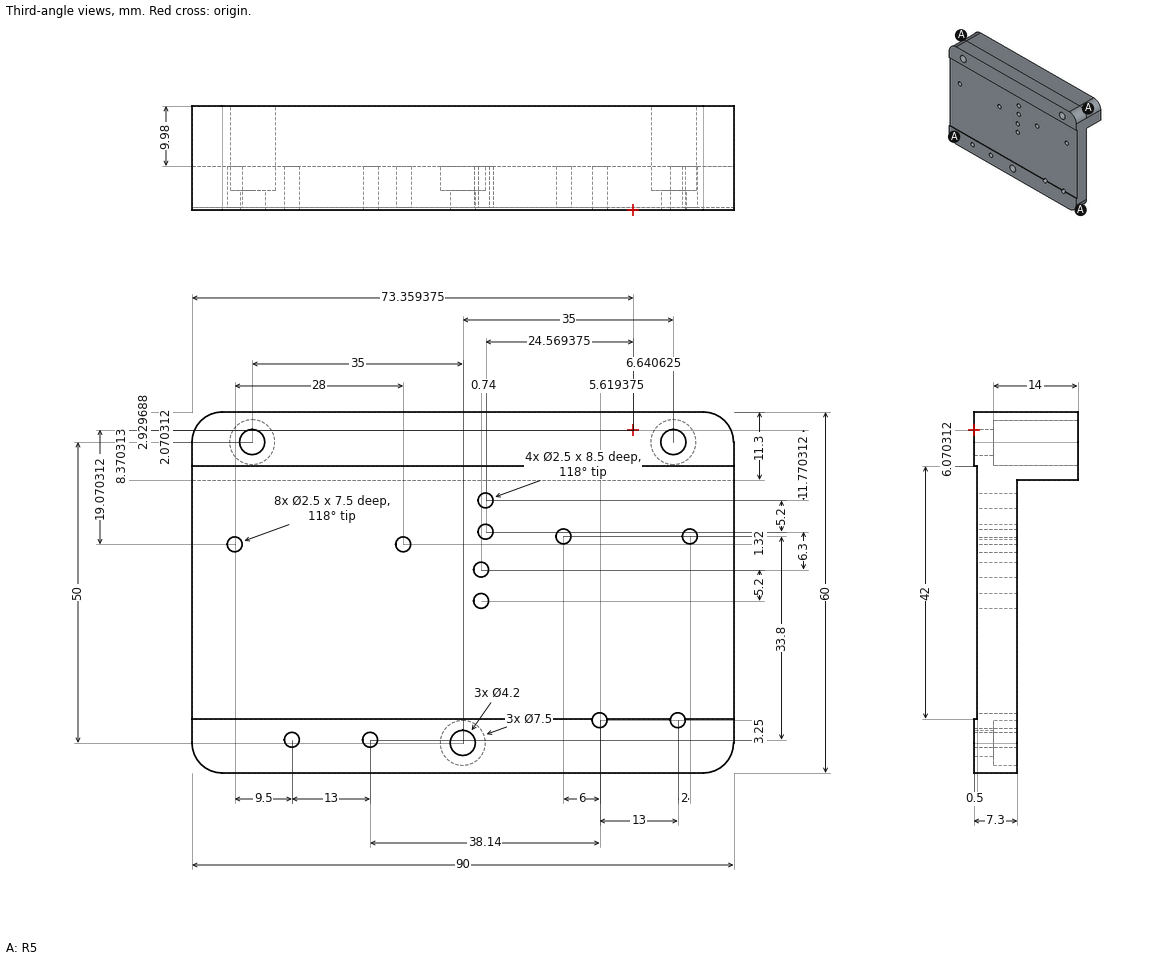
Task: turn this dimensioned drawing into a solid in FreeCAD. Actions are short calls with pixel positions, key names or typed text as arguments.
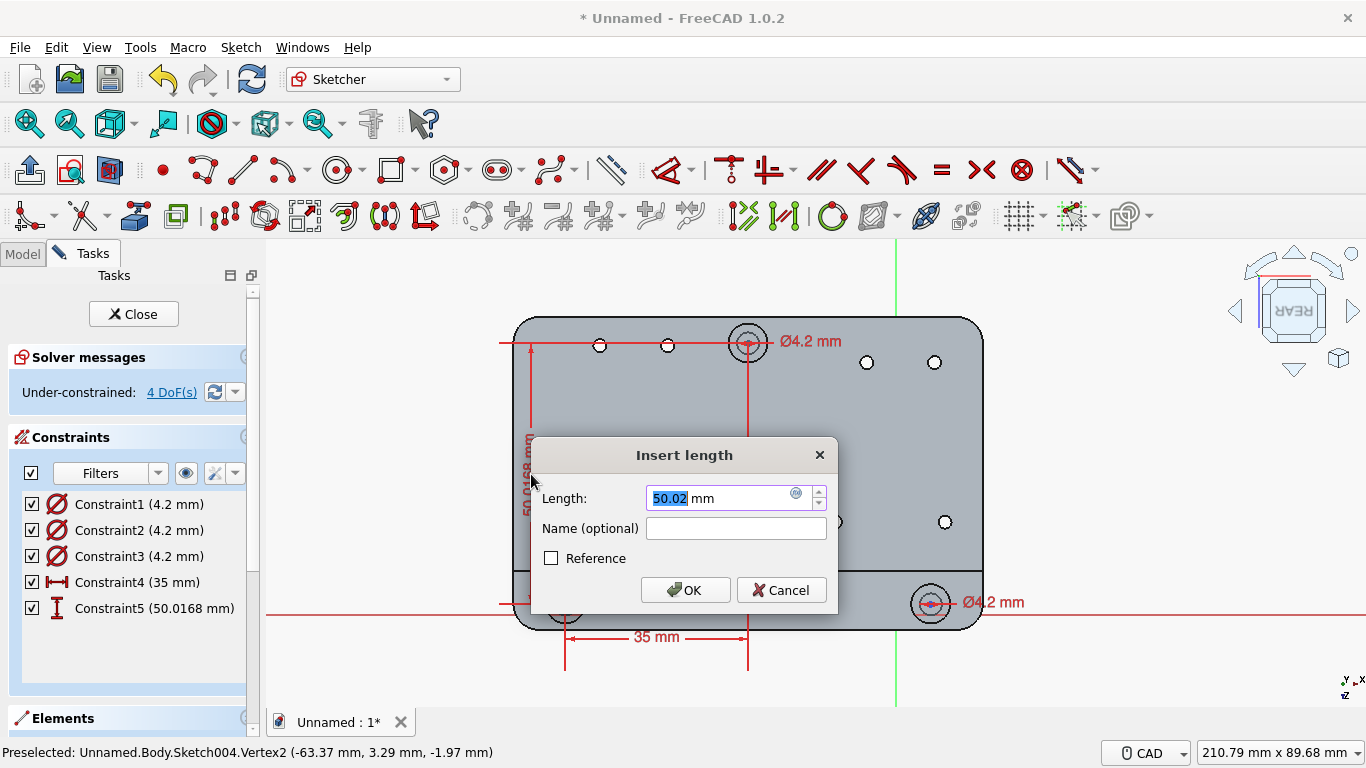
text(50)
key(Return)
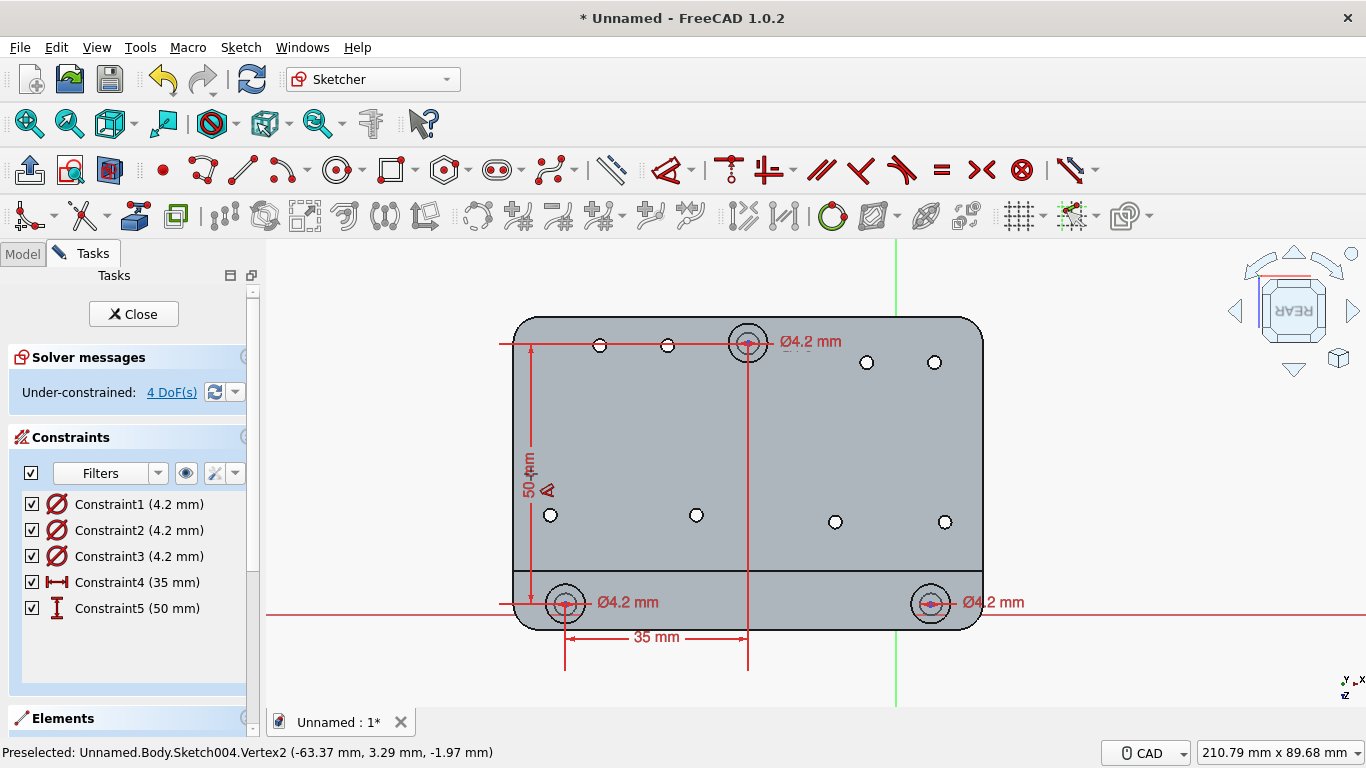
click(748, 344)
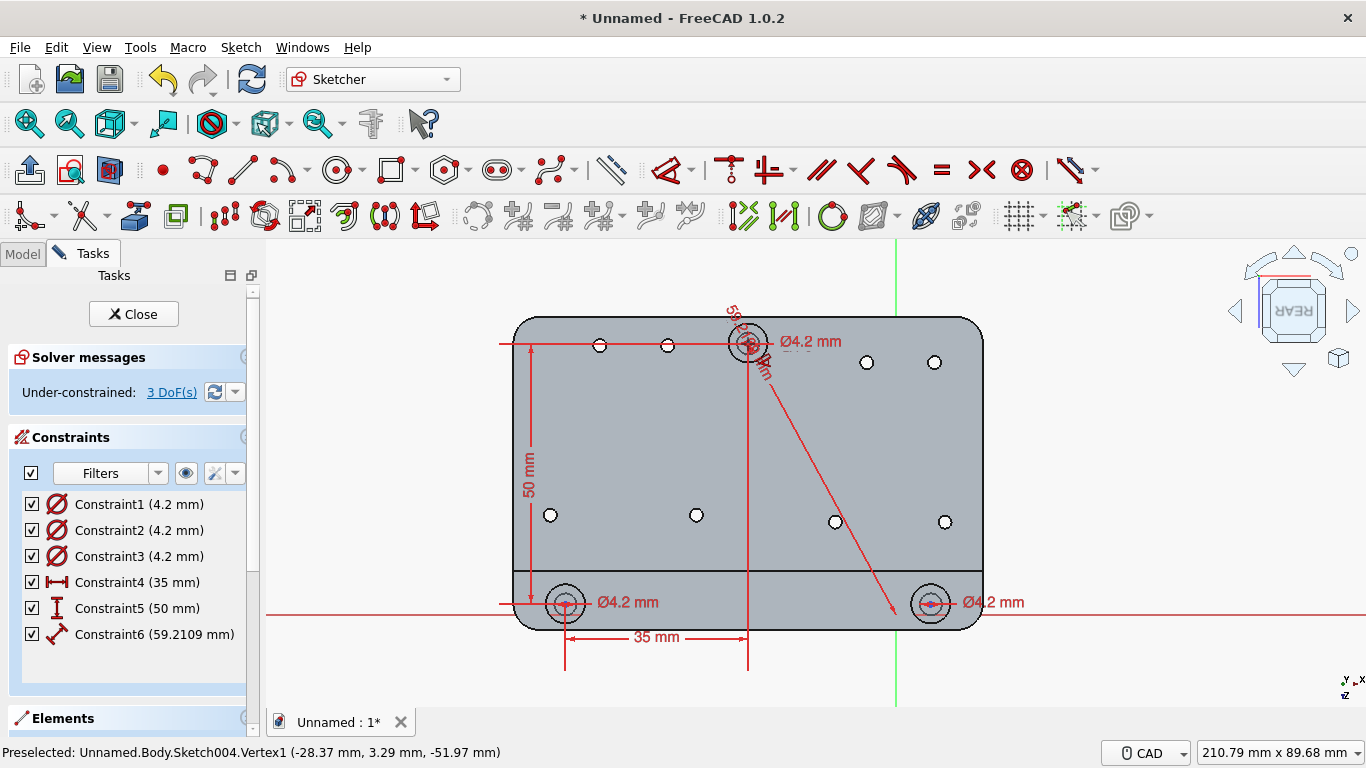
click(931, 604)
click(839, 638)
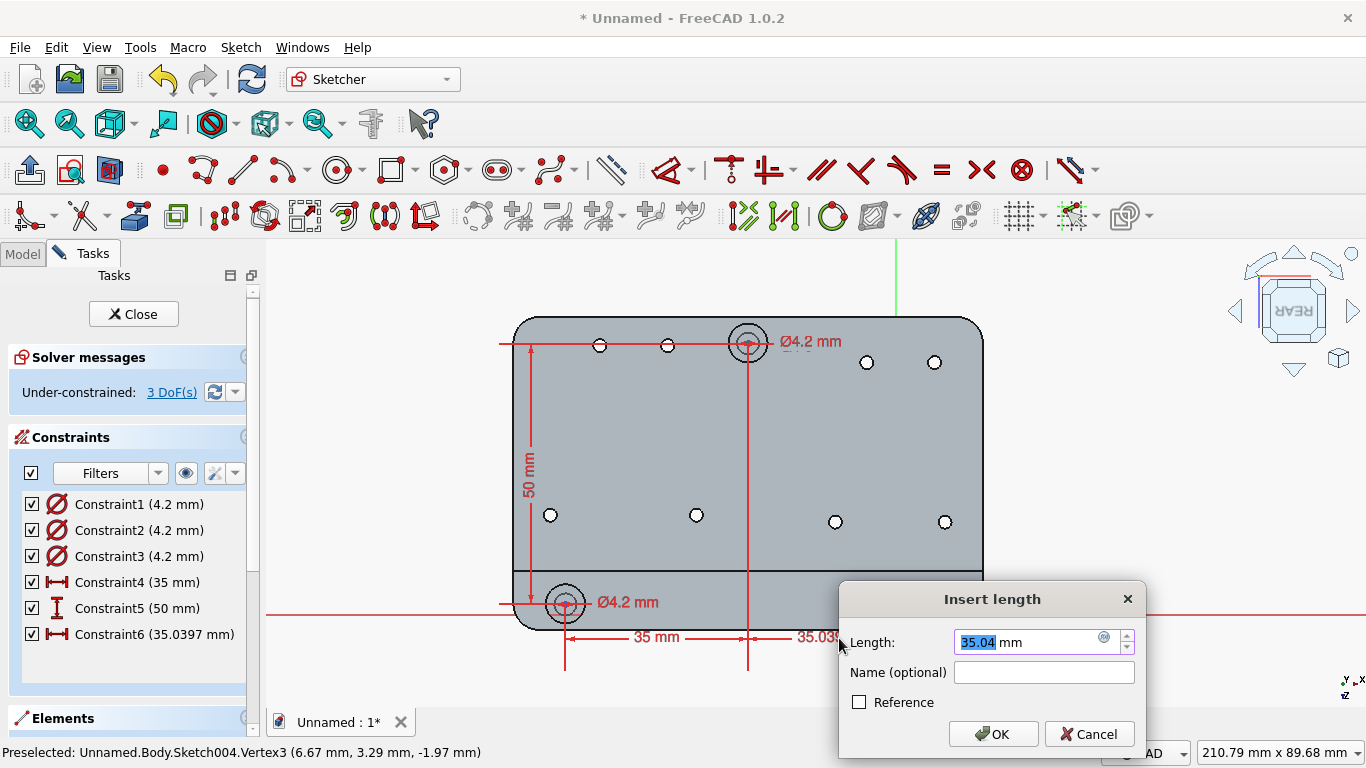
text(35)
key(Return)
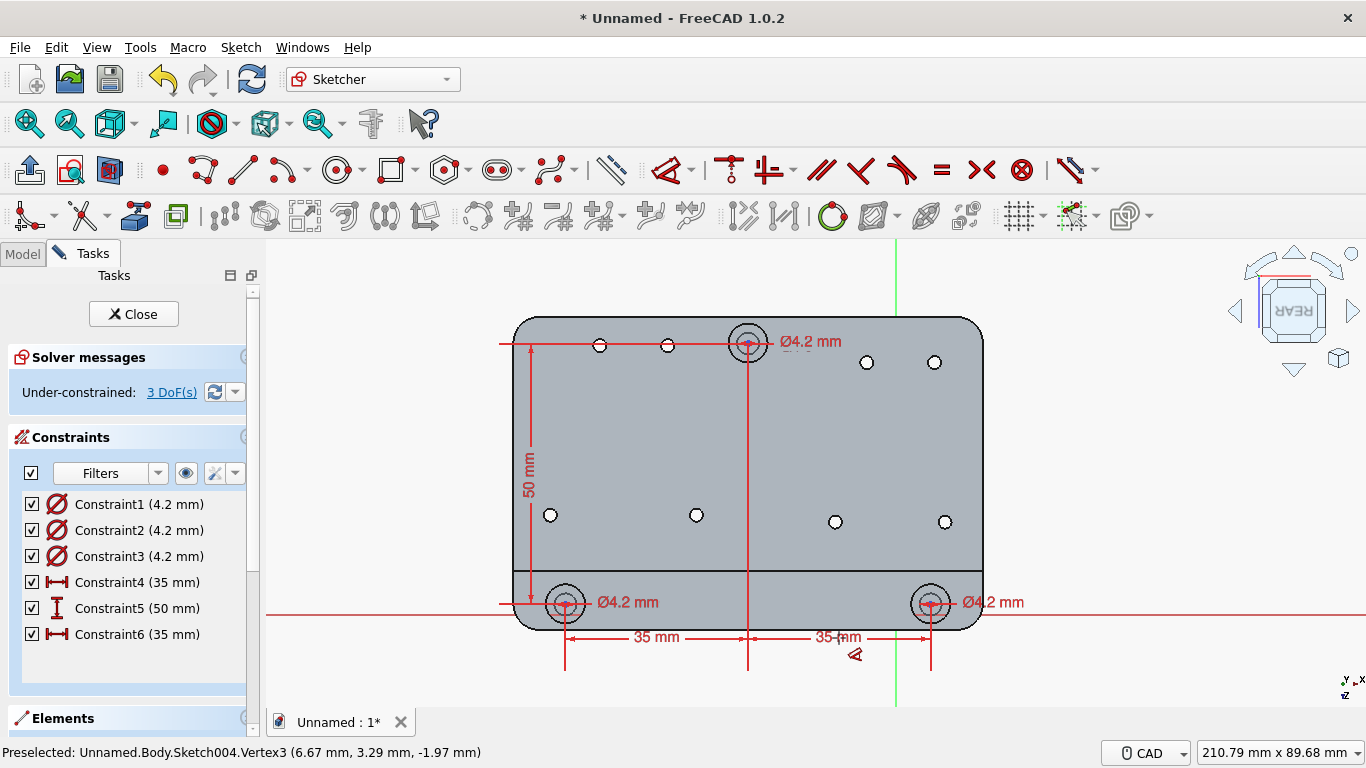
click(748, 344)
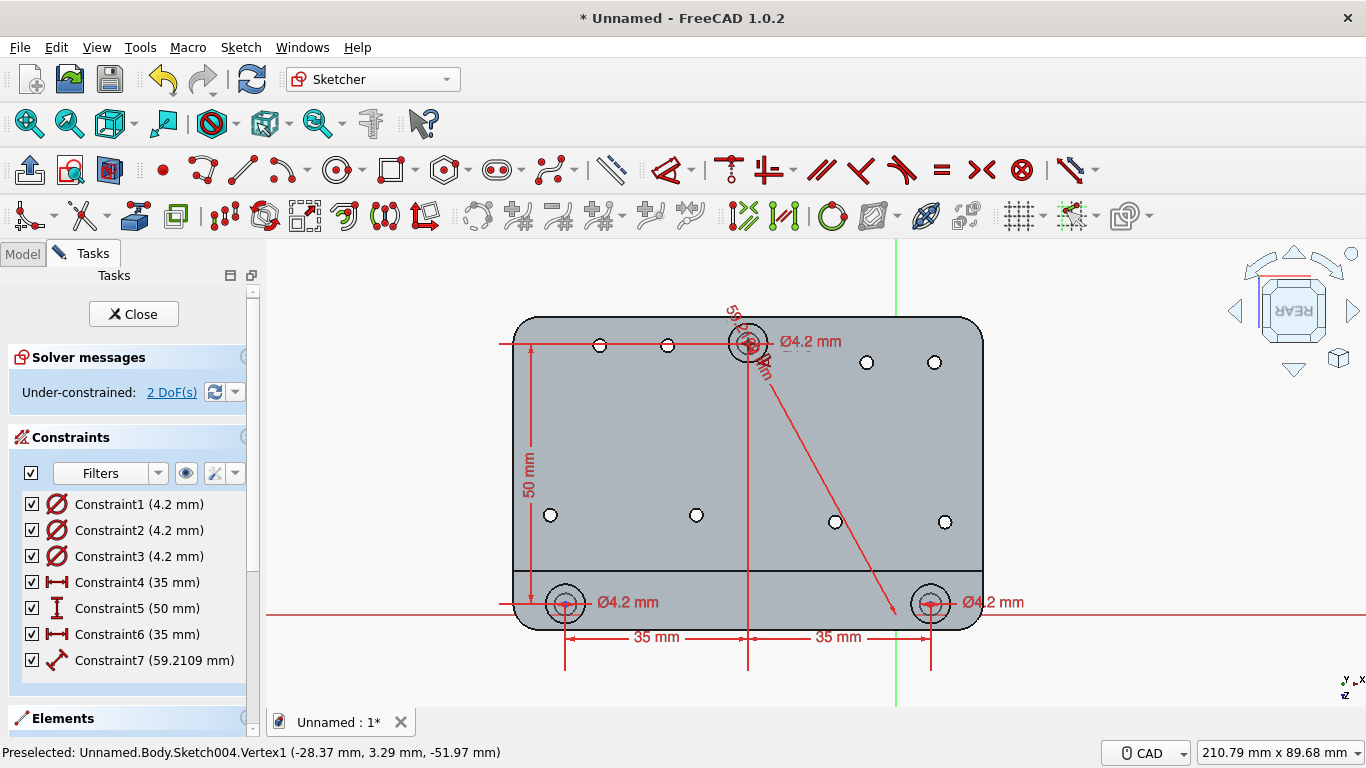
click(931, 604)
click(965, 474)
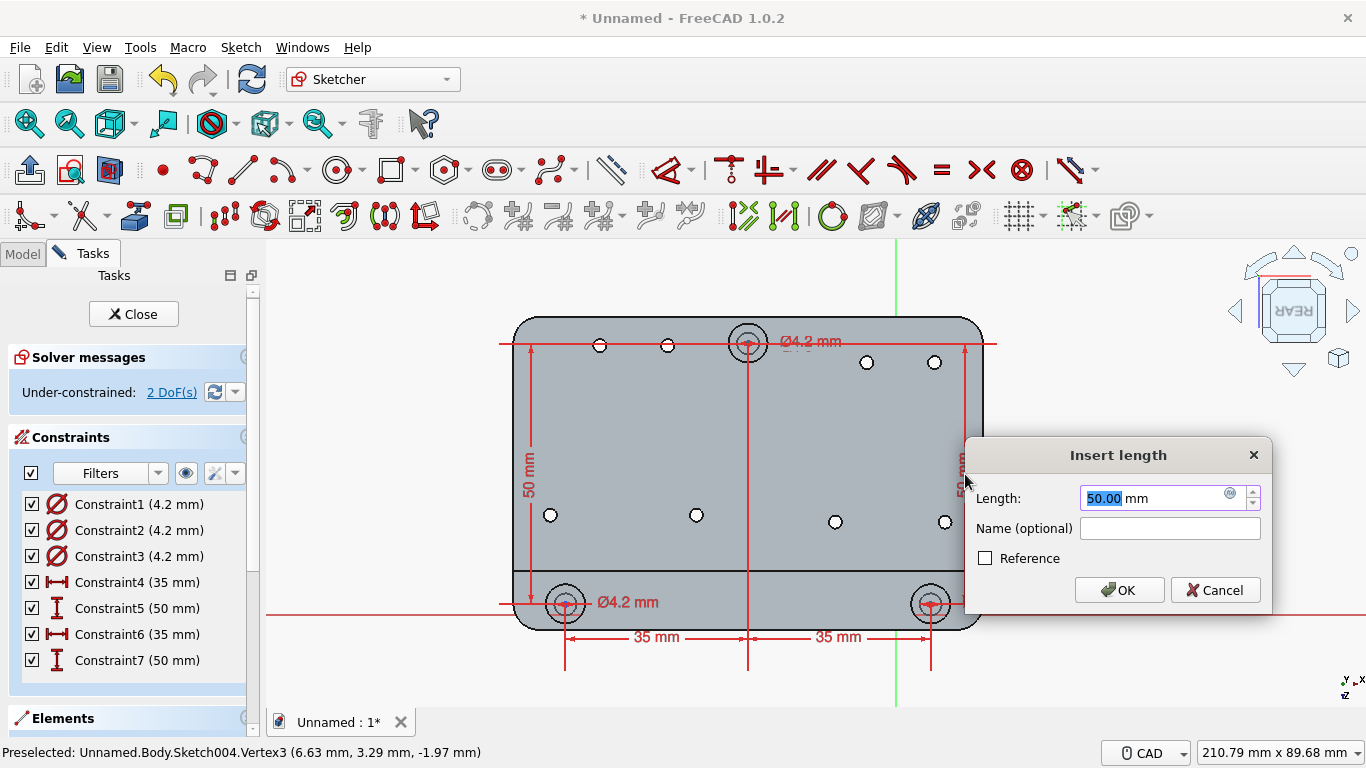
text(50)
key(Return)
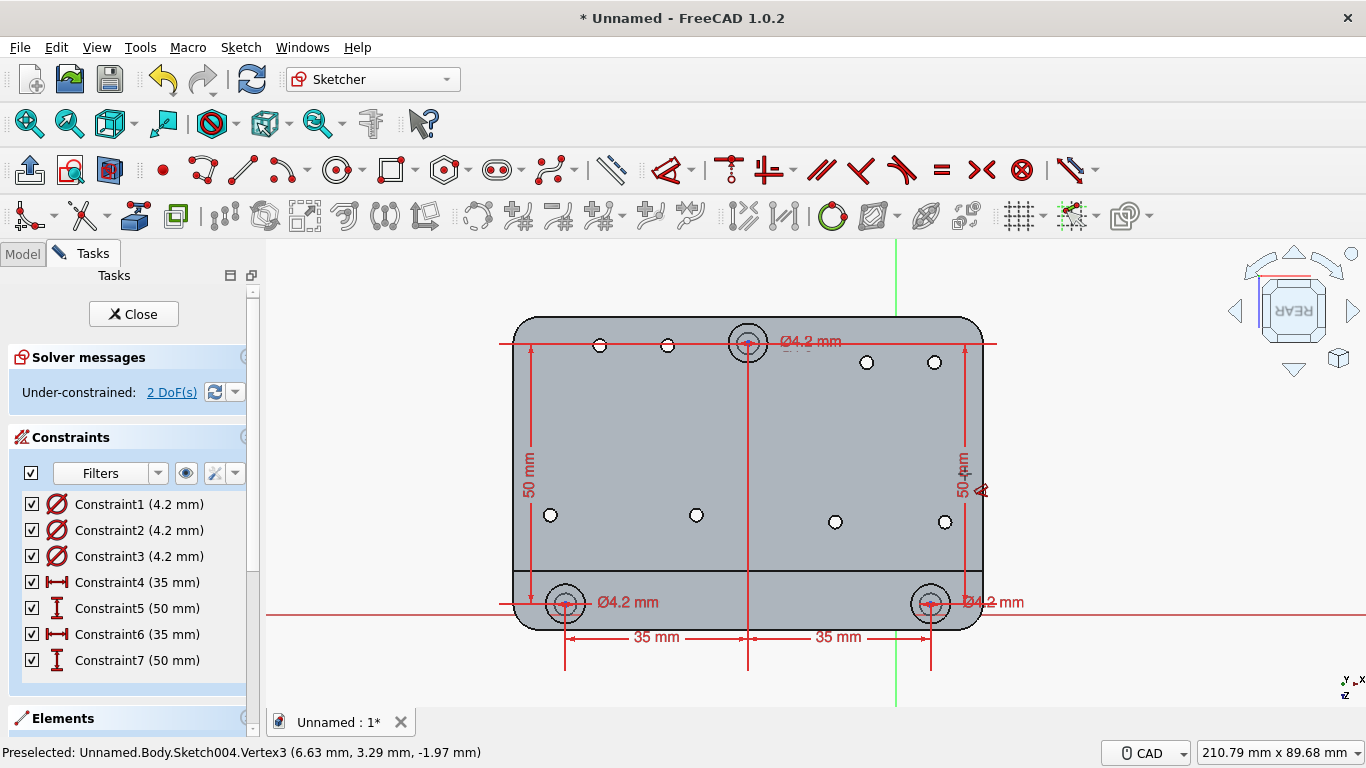
scroll(565, 604, up, 7)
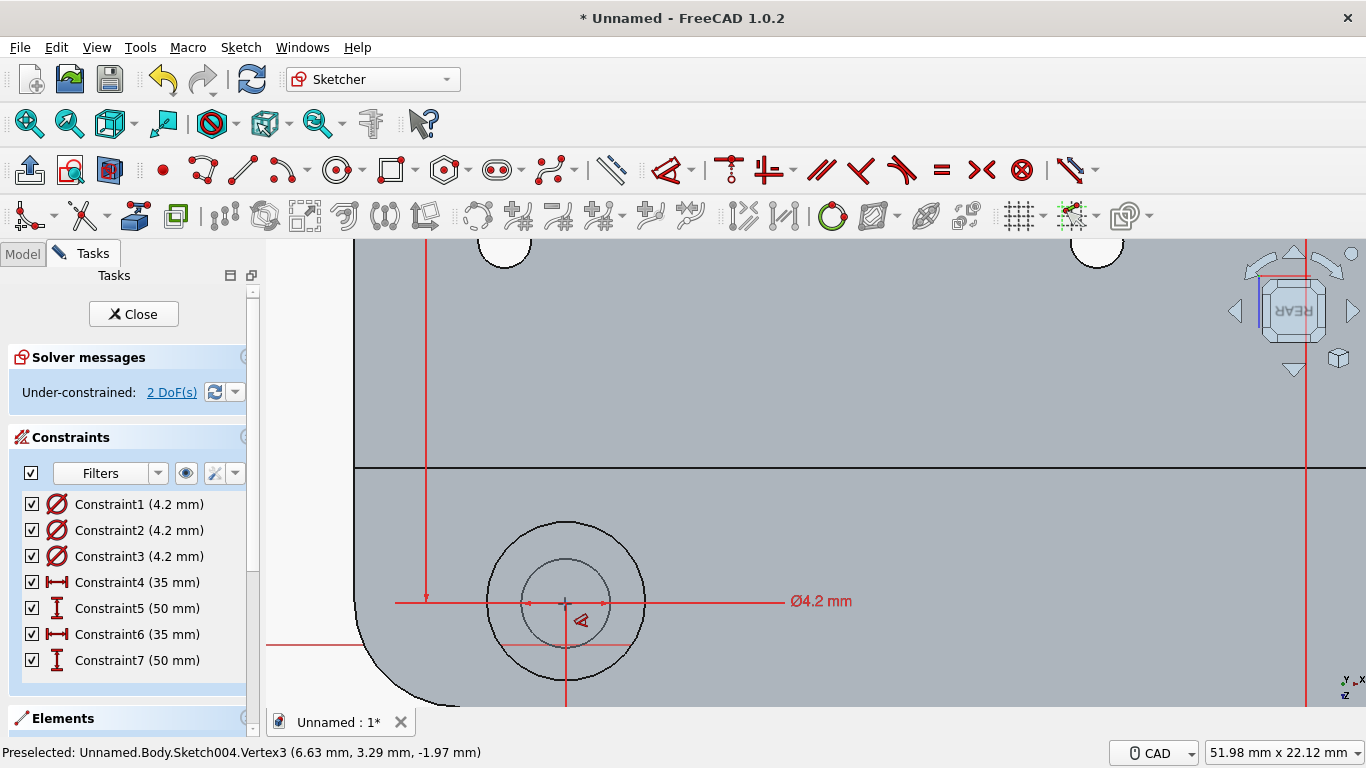
click(566, 603)
click(508, 624)